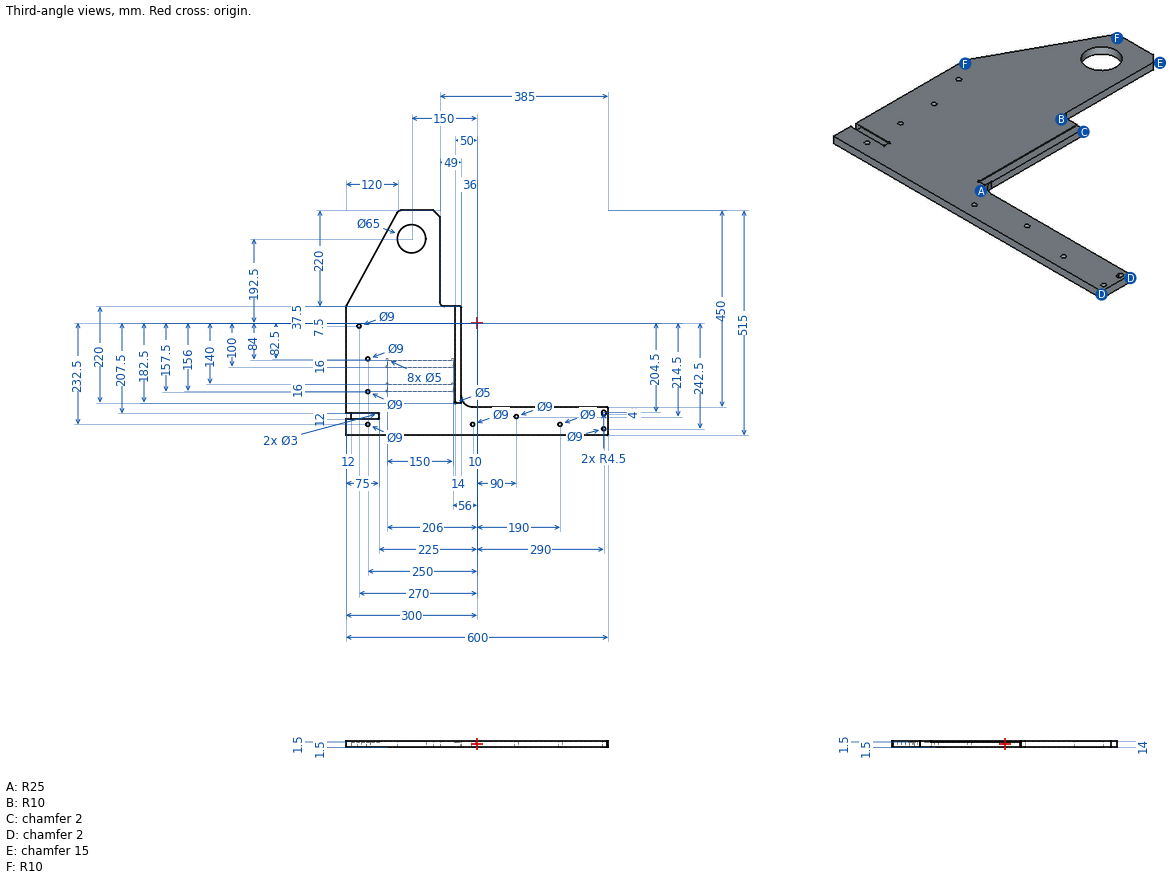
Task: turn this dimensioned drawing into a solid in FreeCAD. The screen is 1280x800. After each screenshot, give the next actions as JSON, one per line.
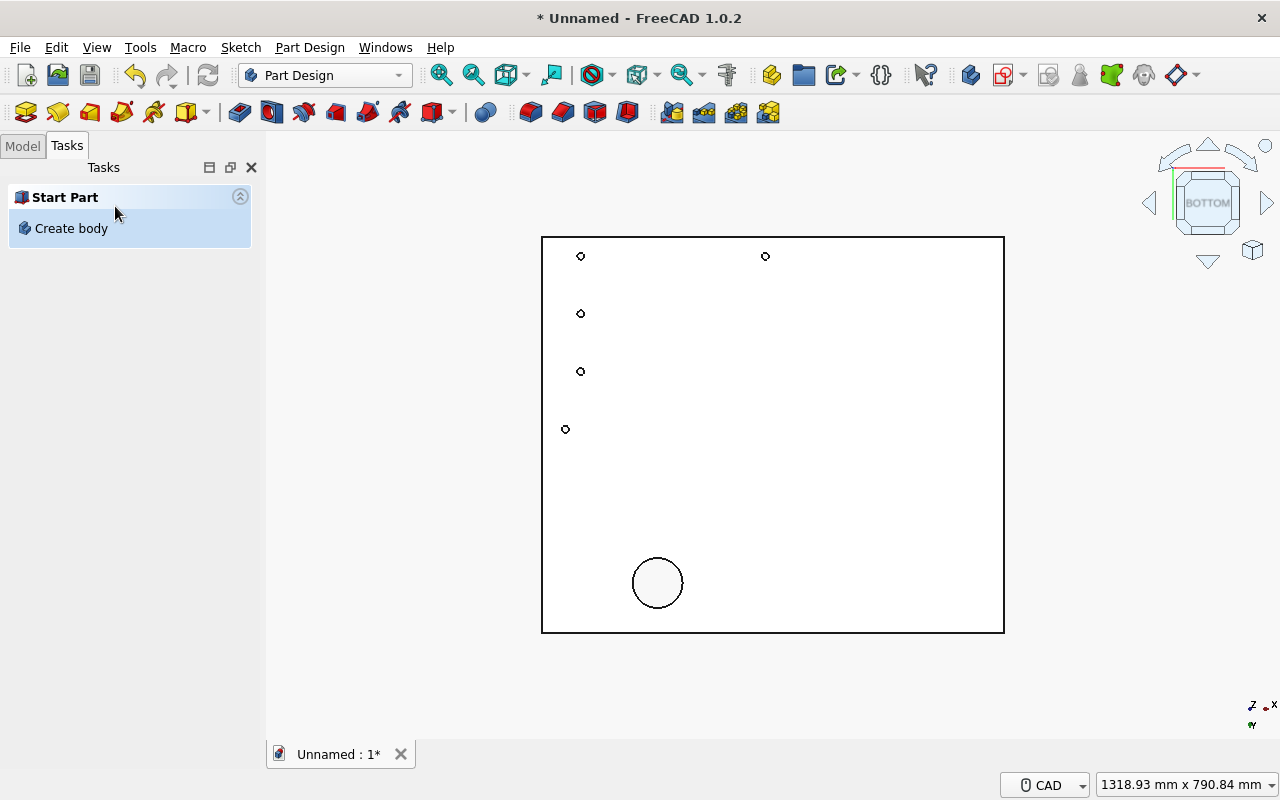
{"action": "left_click", "coordinate": [839, 434]}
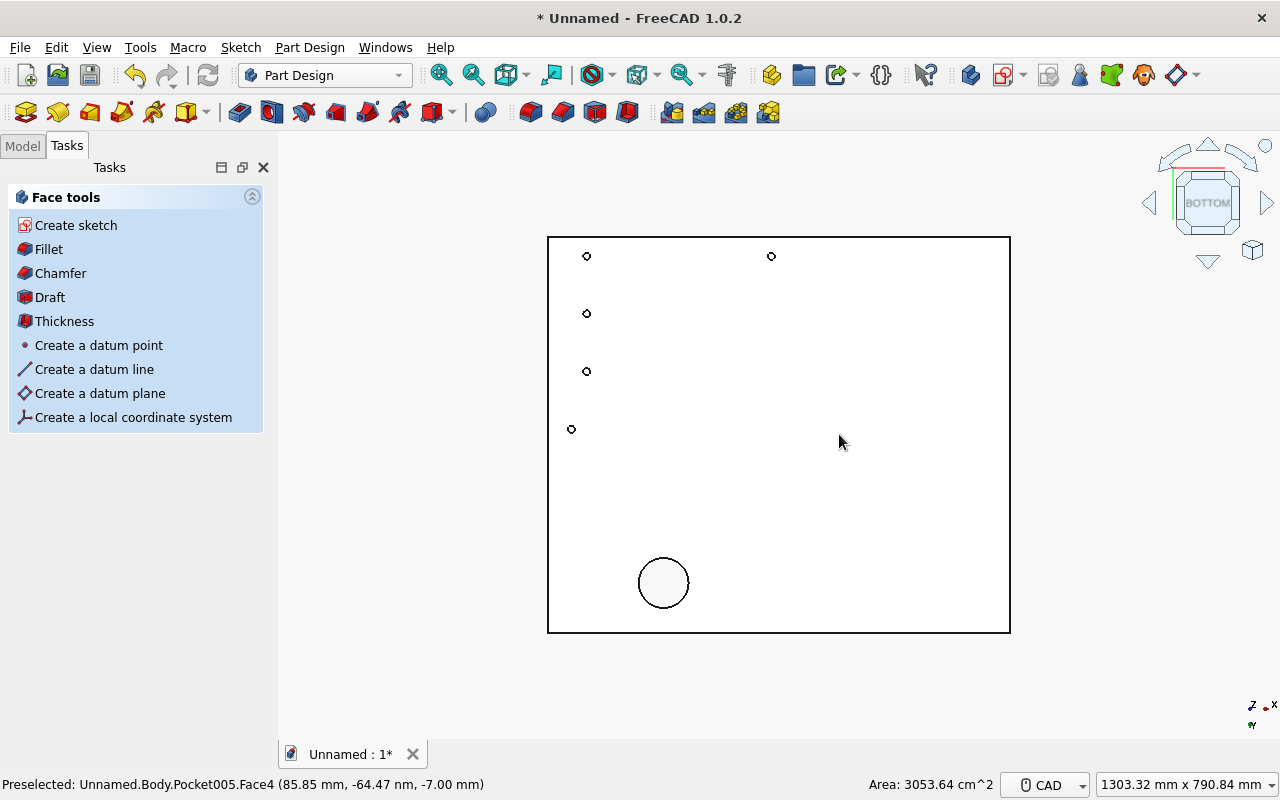
{"action": "left_click", "coordinate": [1004, 76]}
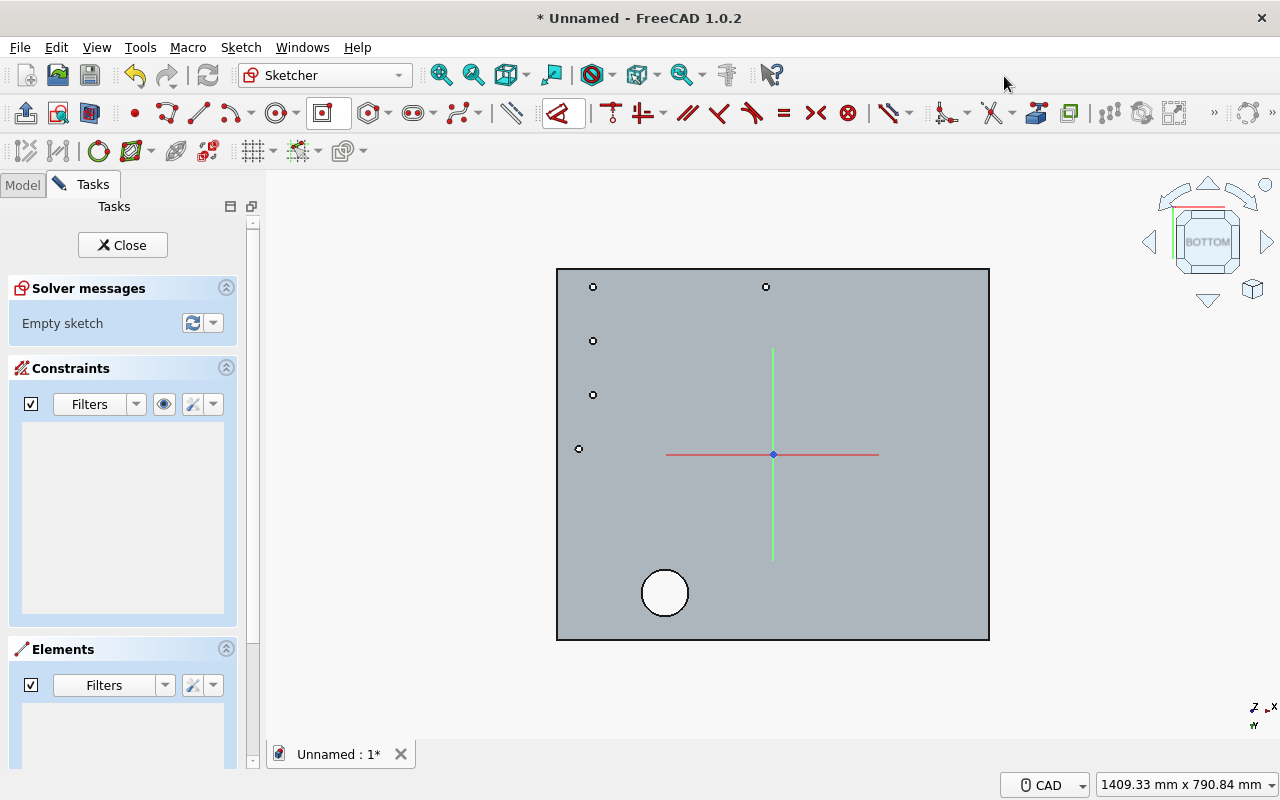
{"action": "scroll", "coordinate": [696, 374], "scroll_direction": "up", "scroll_amount": 6}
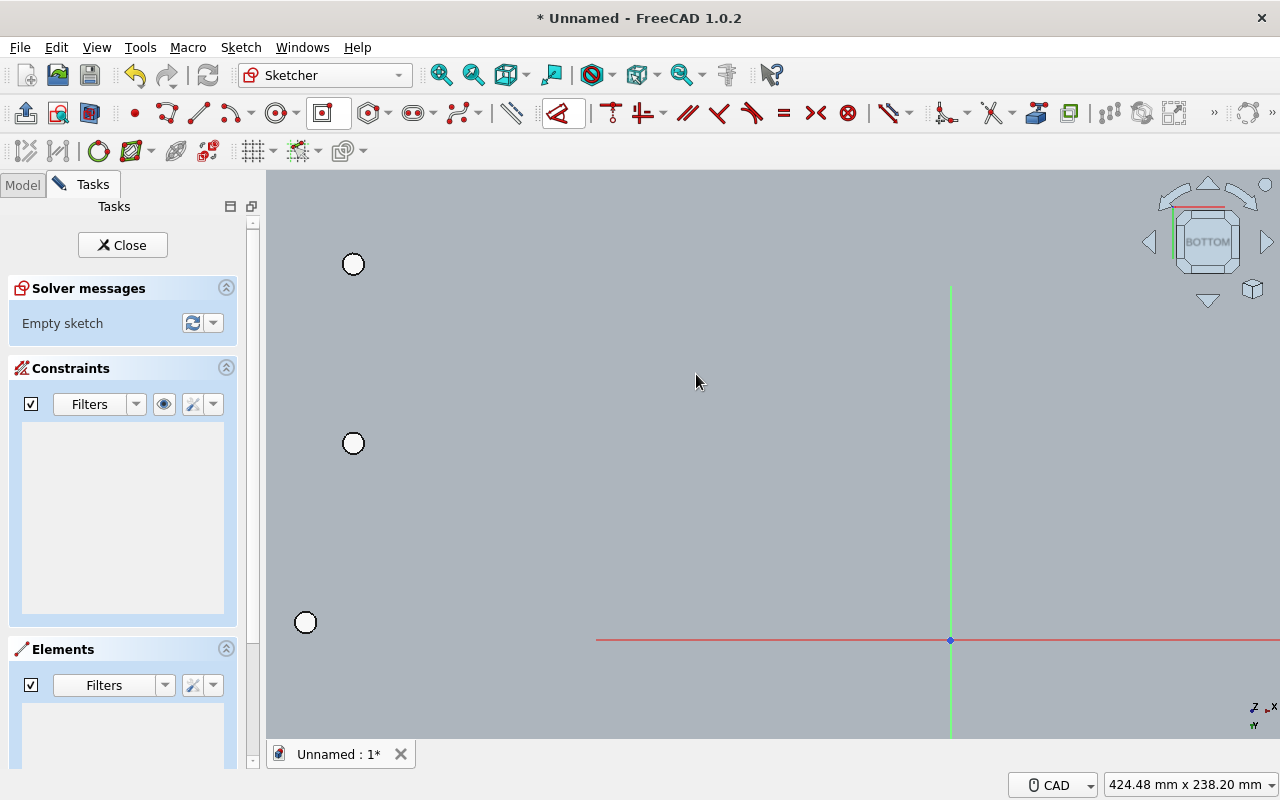
{"action": "key", "text": "g r"}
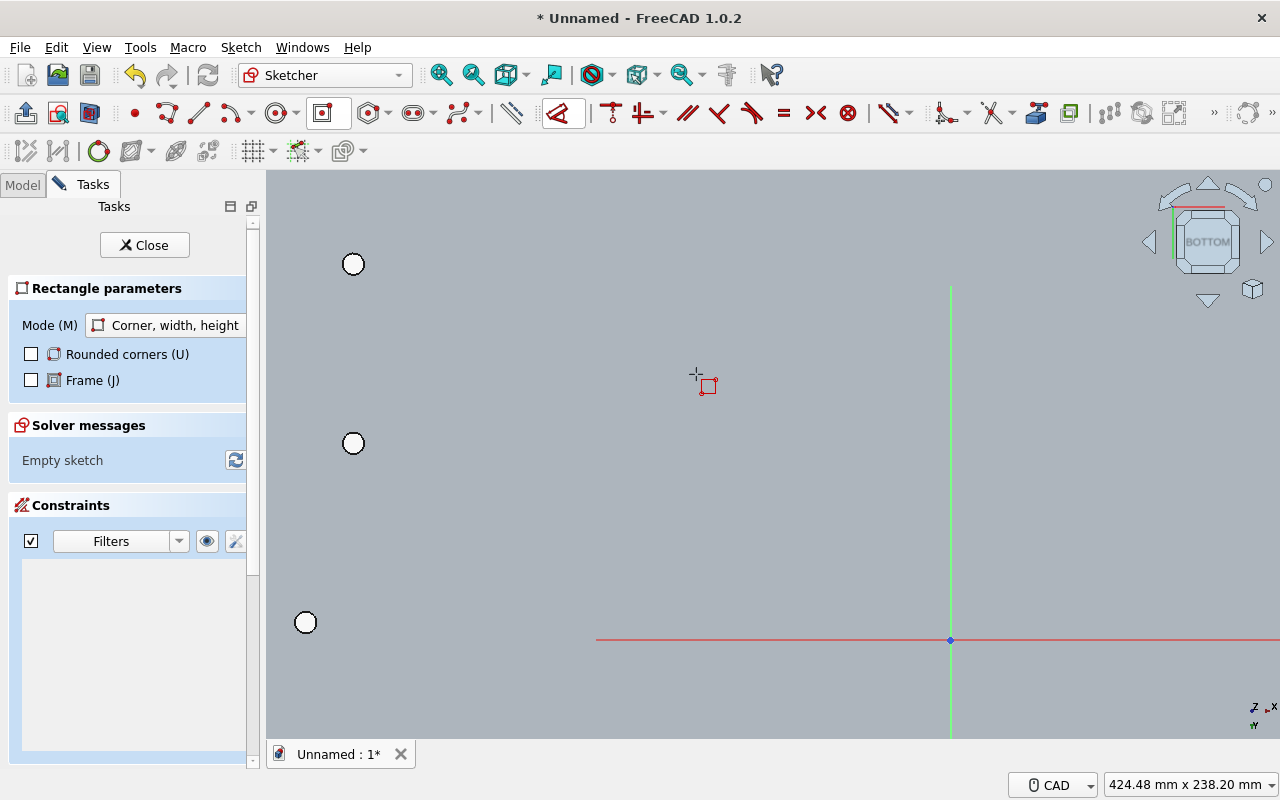
{"action": "left_click", "coordinate": [459, 402]}
{"action": "mouse_move", "coordinate": [817, 440]}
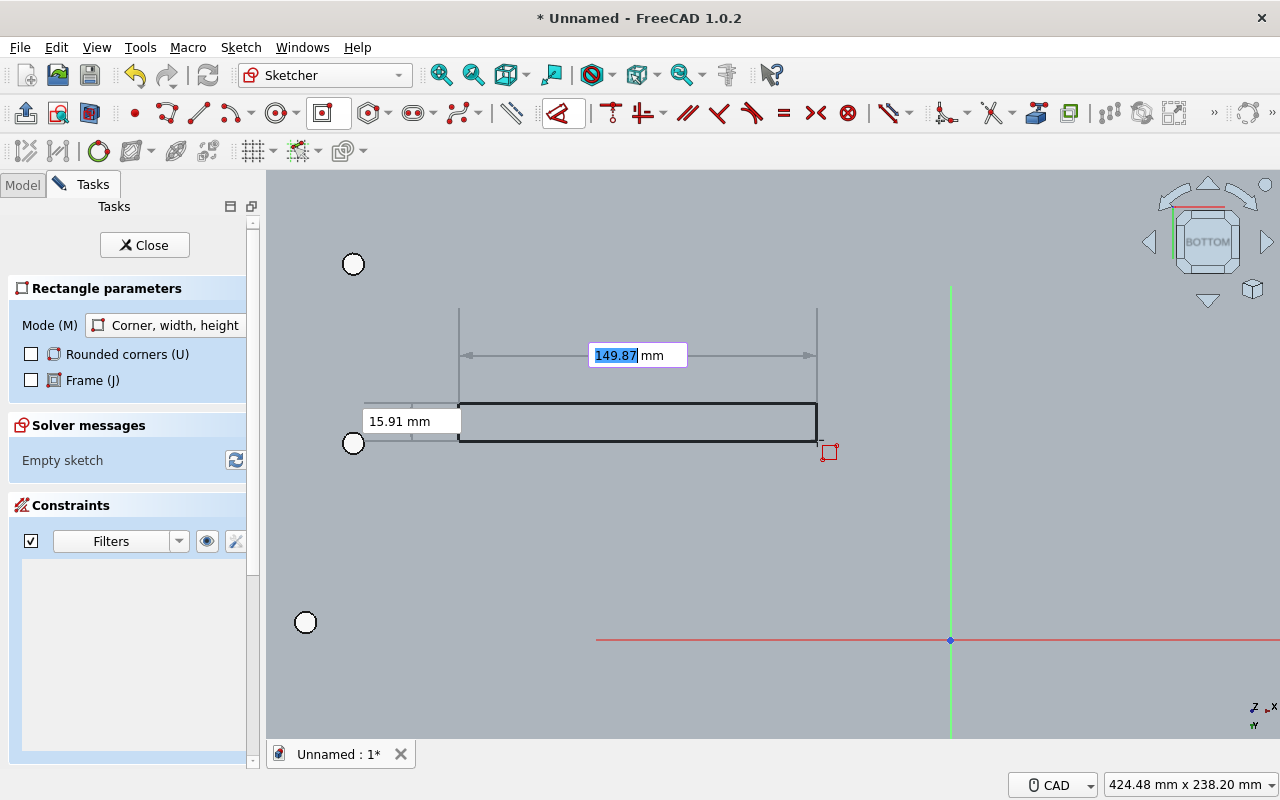
{"action": "type", "text": "150"}
{"action": "key", "text": "Tab"}
{"action": "type", "text": "16"}
{"action": "key", "text": "Return"}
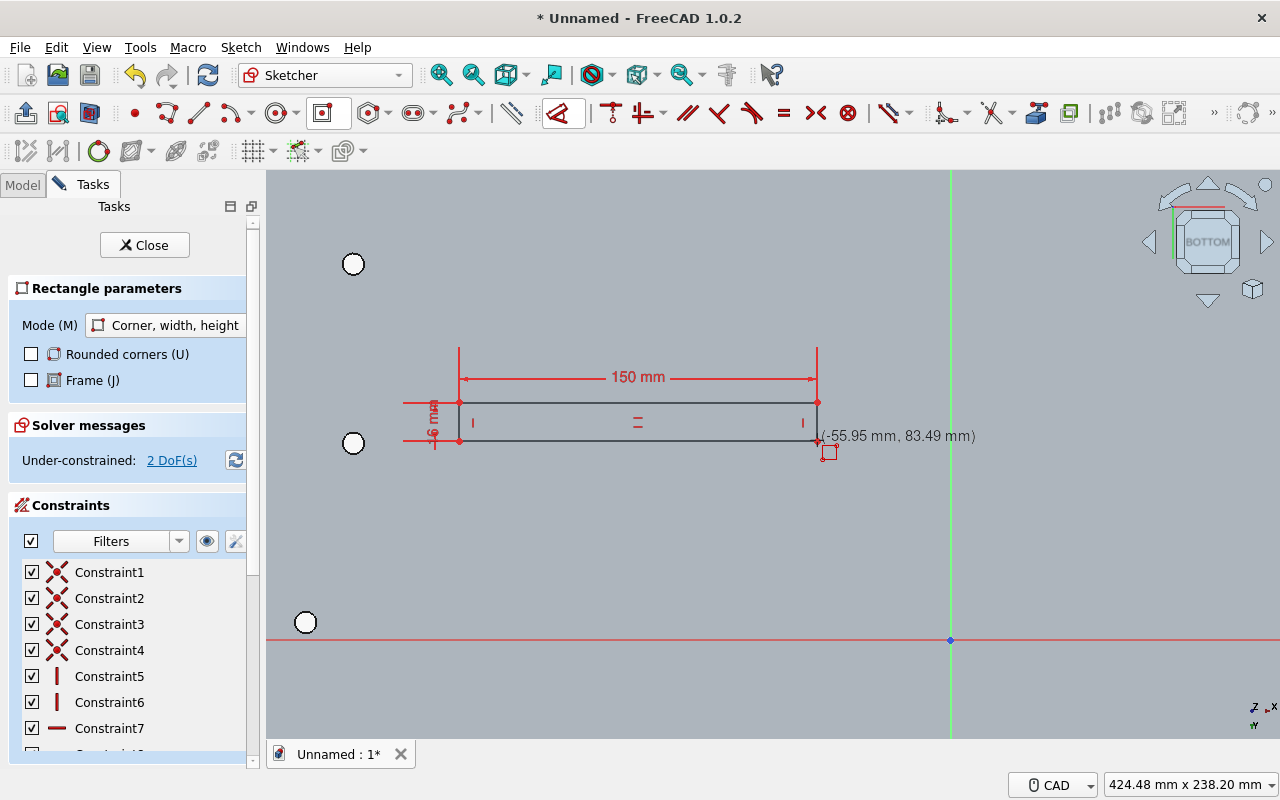
{"action": "left_click", "coordinate": [459, 268]}
{"action": "mouse_move", "coordinate": [817, 306]}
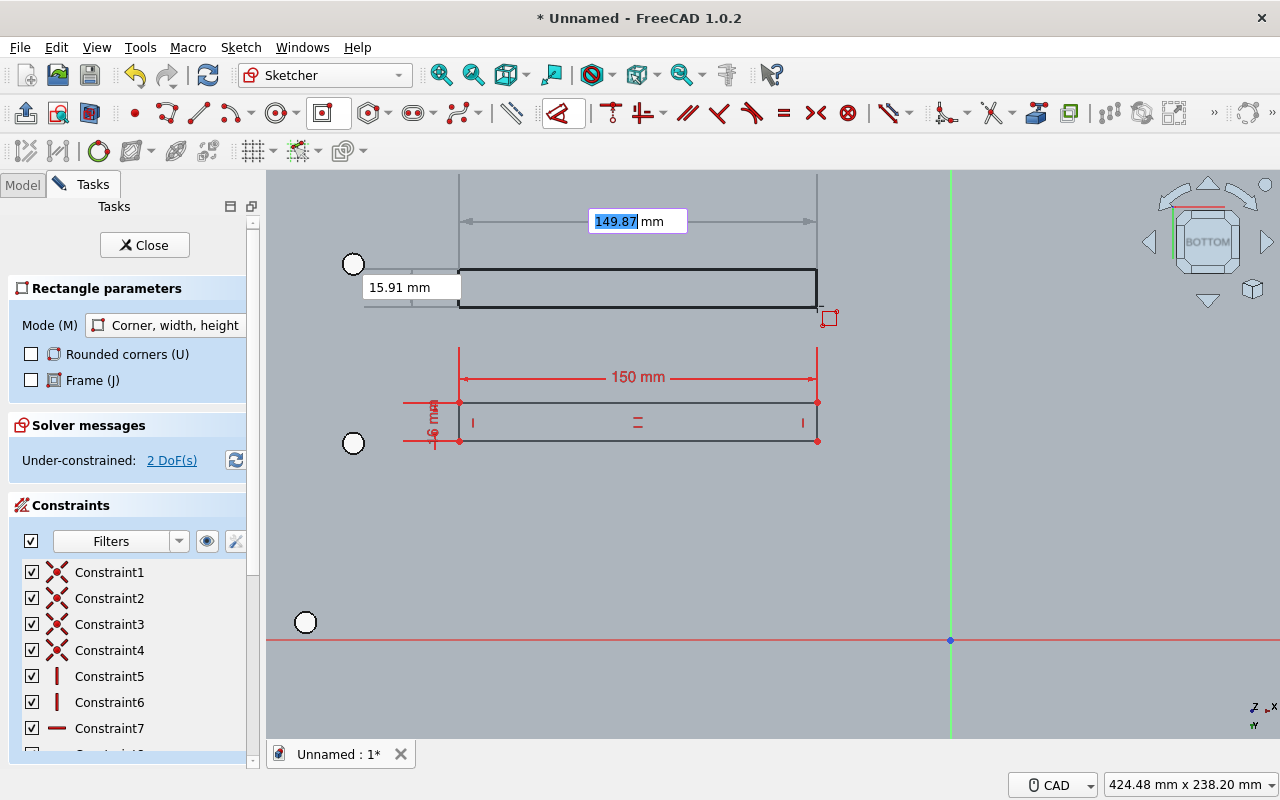
{"action": "type", "text": "150"}
{"action": "key", "text": "Tab"}
{"action": "type", "text": "16"}
{"action": "key", "text": "Return"}
{"action": "key", "text": "Escape"}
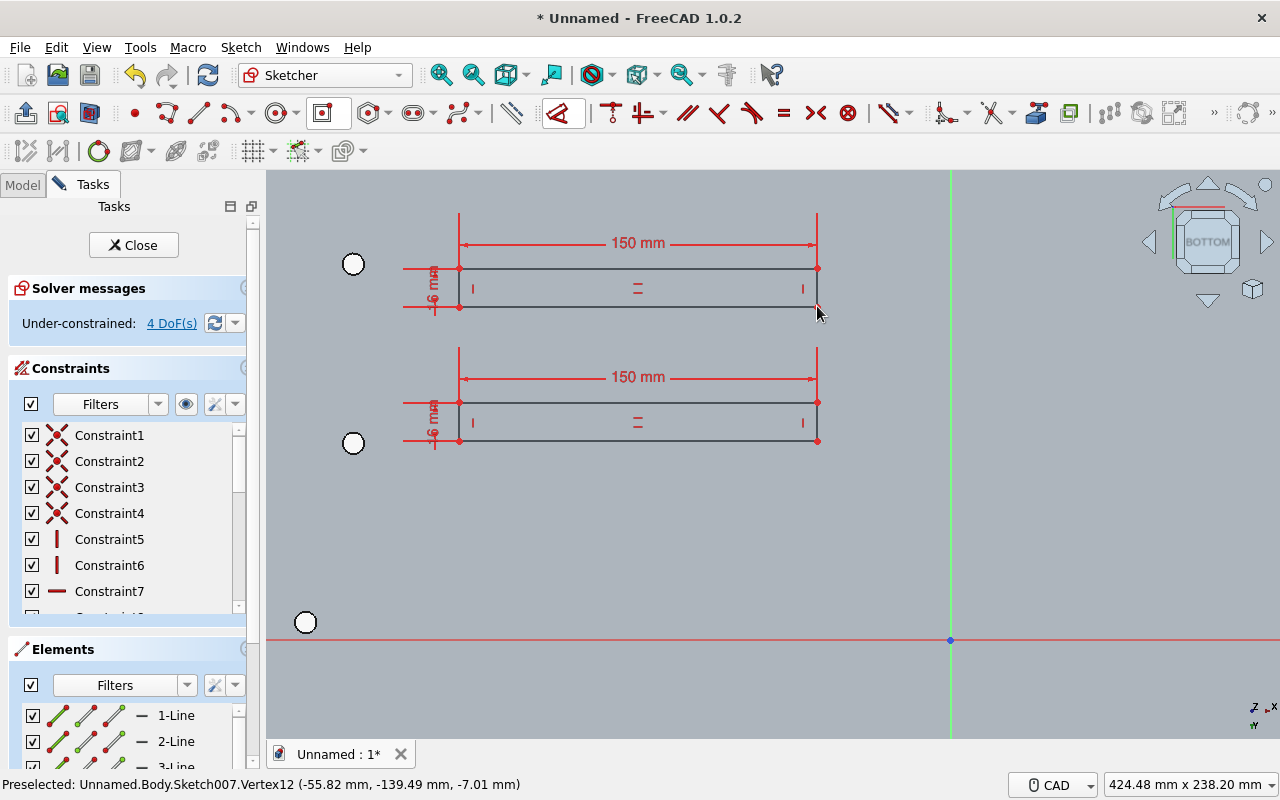
{"action": "left_click", "coordinate": [459, 441]}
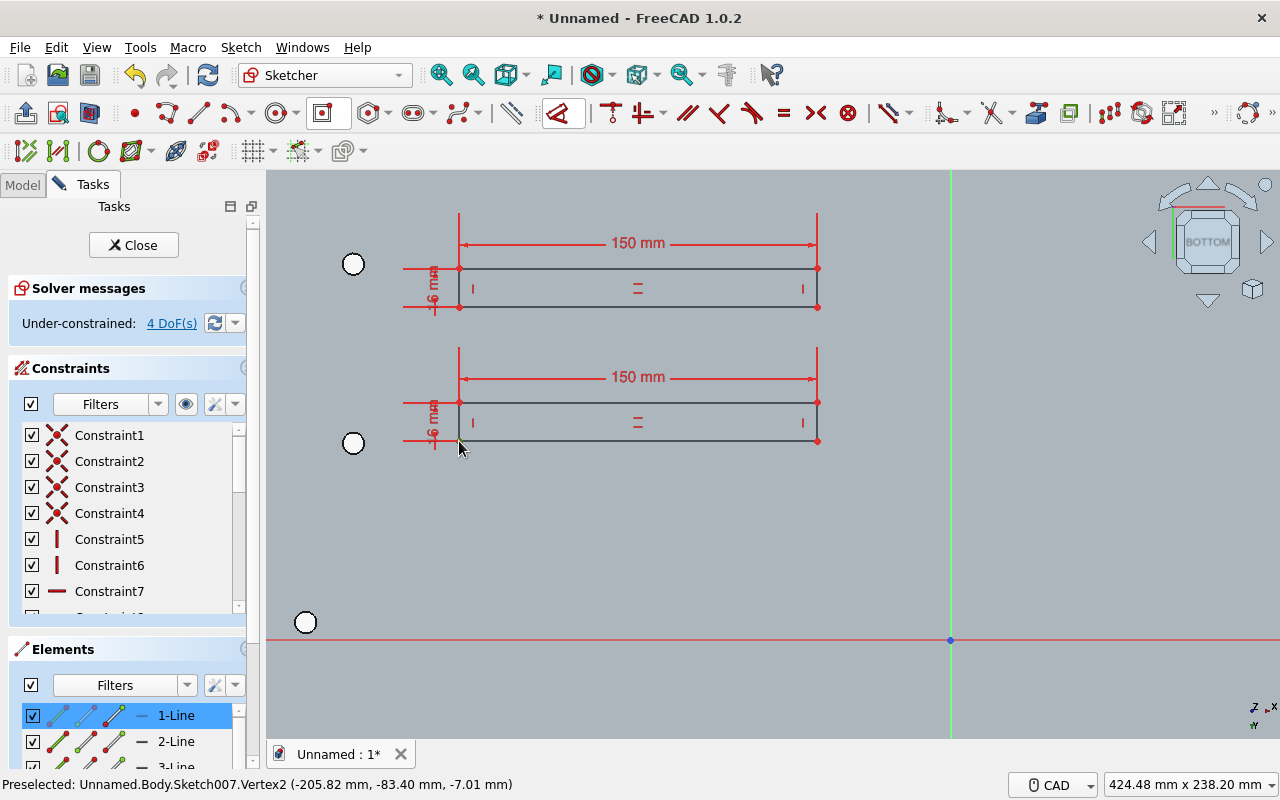
{"action": "key", "text": "i"}